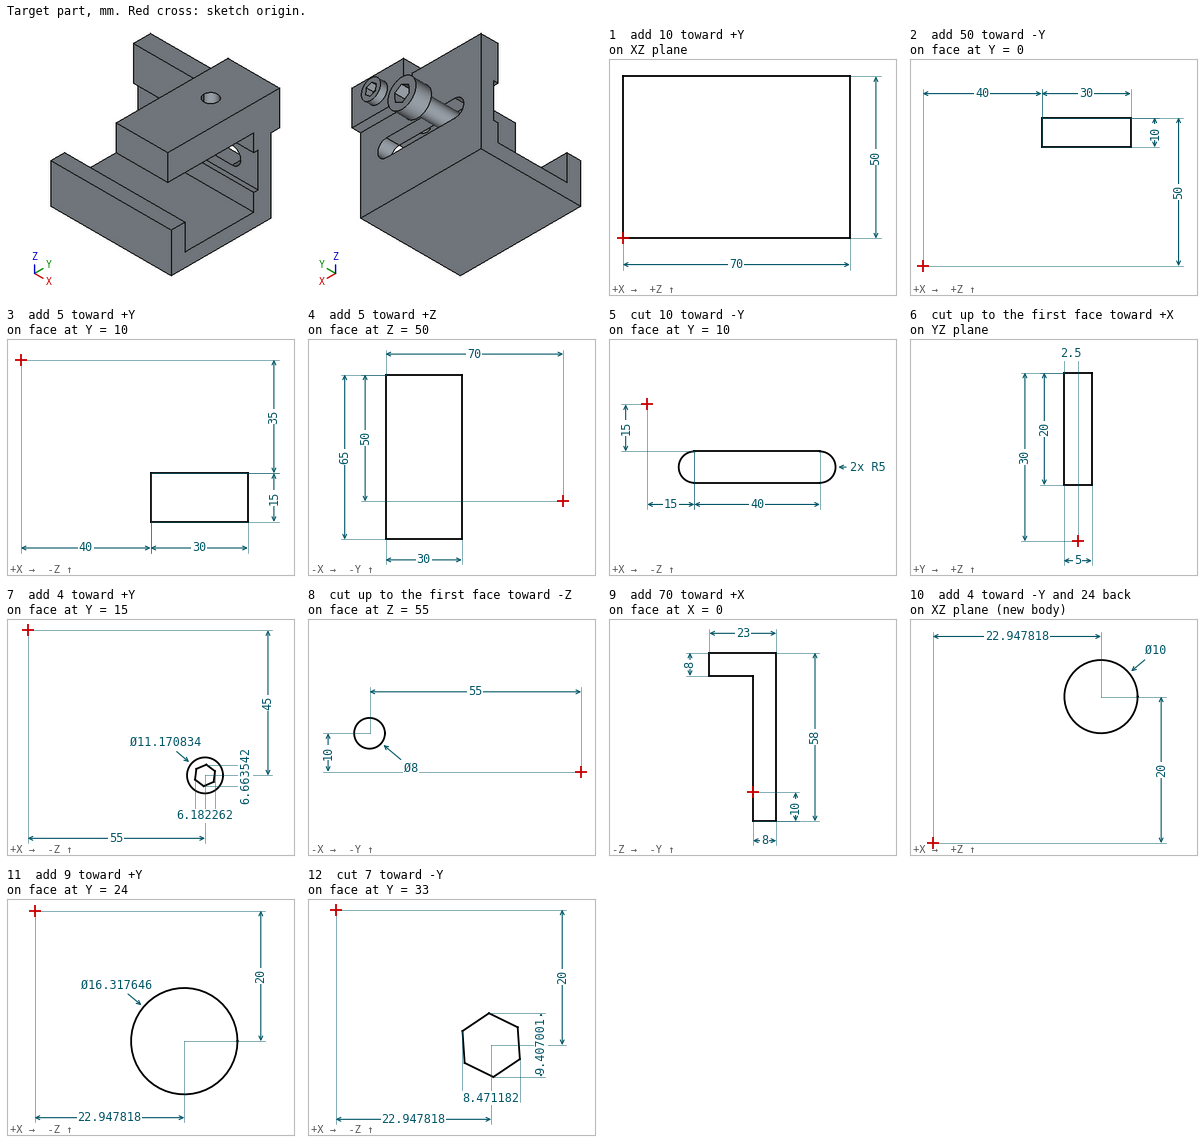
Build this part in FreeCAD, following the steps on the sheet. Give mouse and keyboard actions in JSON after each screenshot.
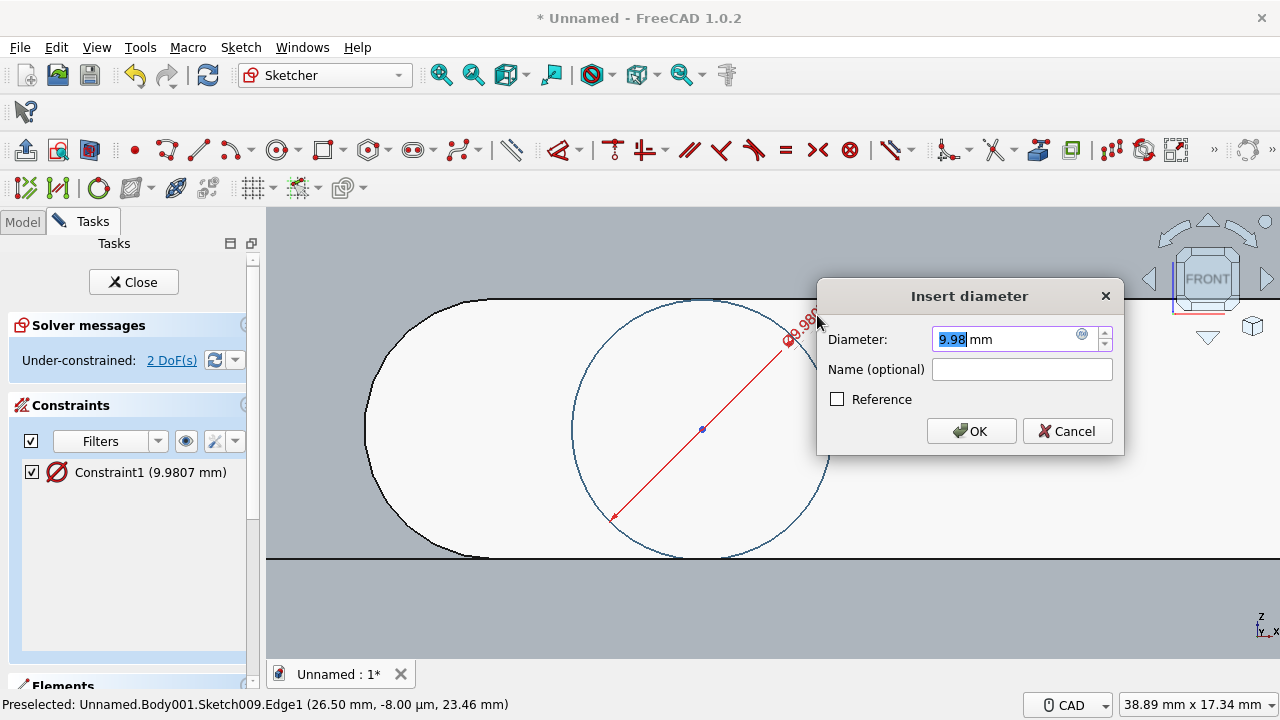
{"action": "type", "text": "10"}
{"action": "key", "text": "Return"}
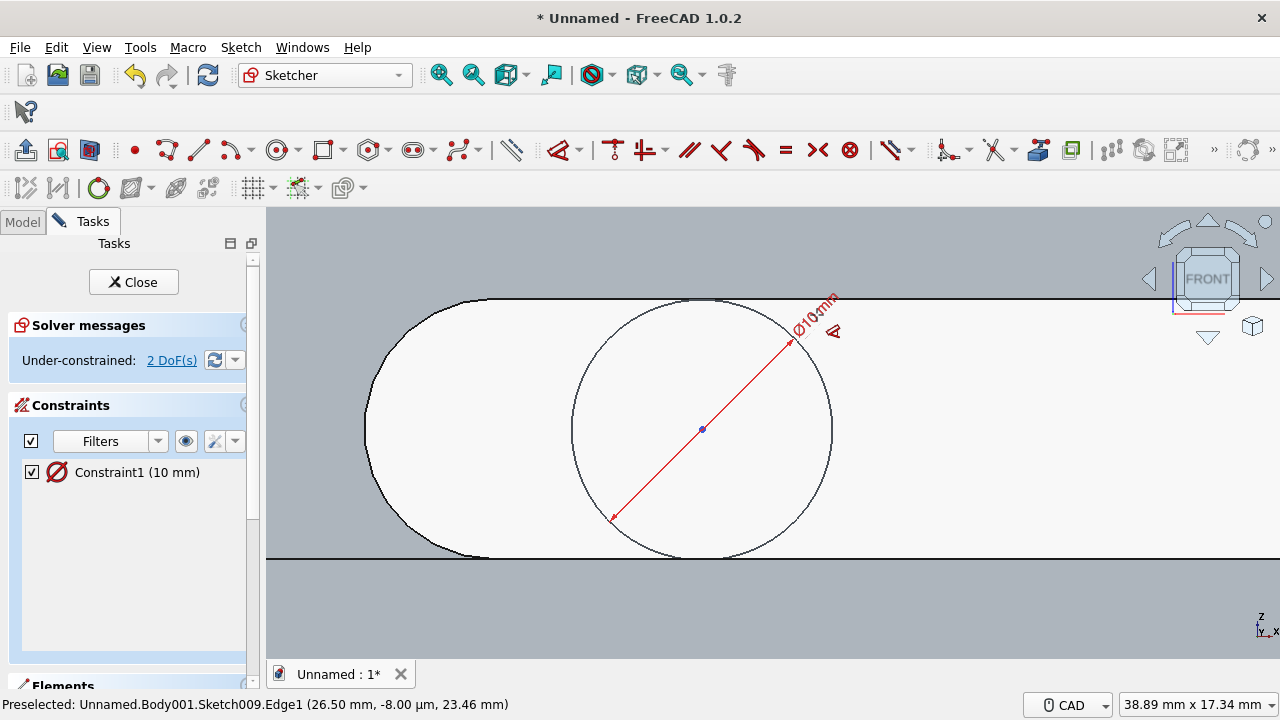
{"action": "left_click", "coordinate": [702, 430]}
{"action": "left_click", "coordinate": [736, 531]}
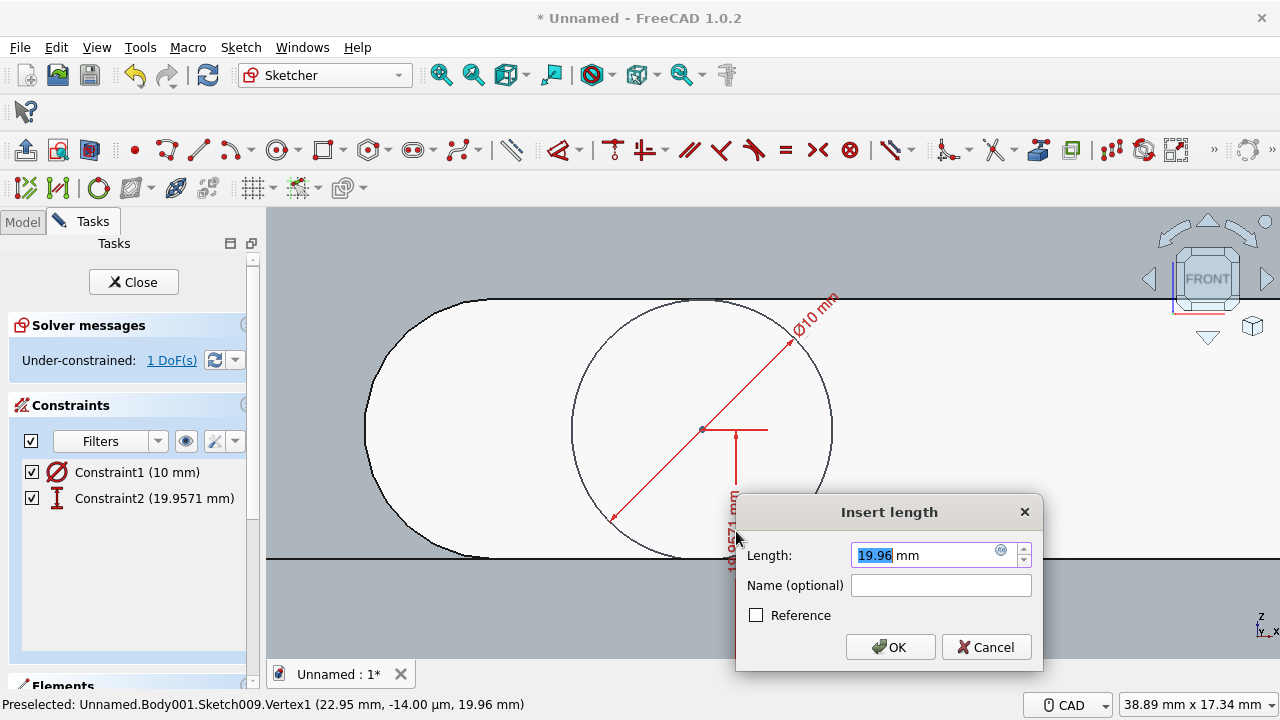
{"action": "type", "text": "20"}
{"action": "key", "text": "Return"}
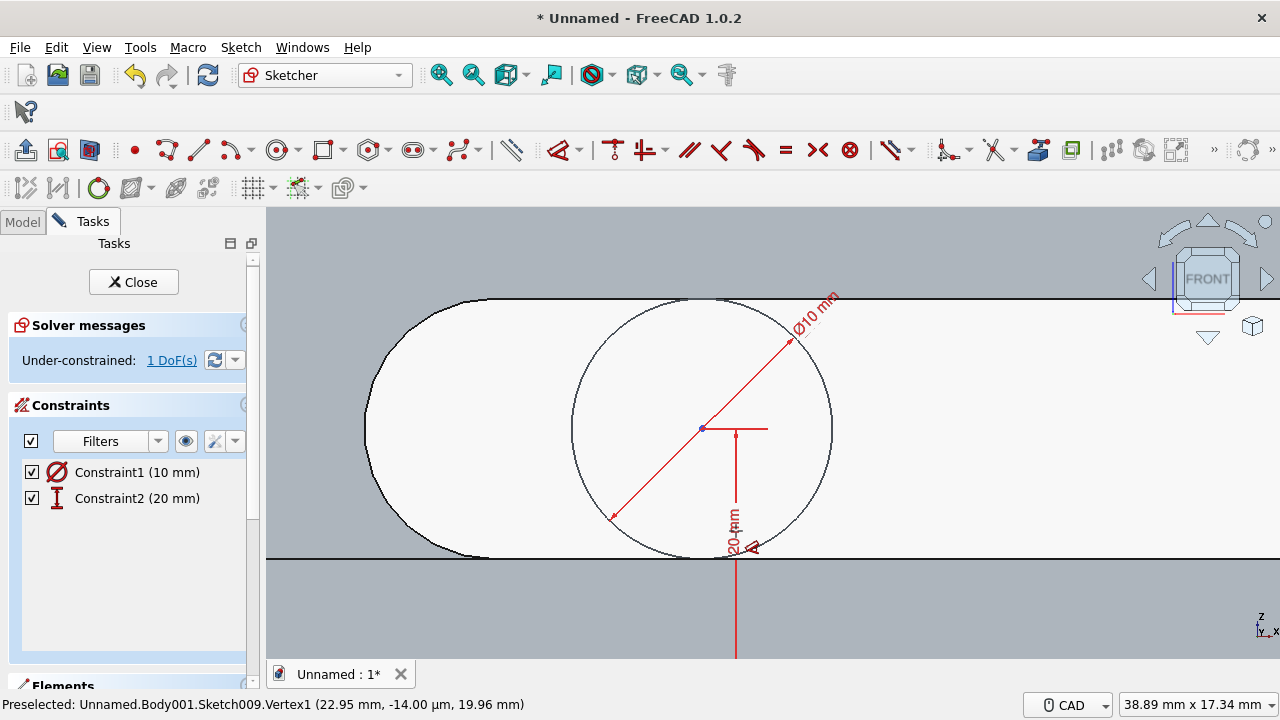
{"action": "left_click", "coordinate": [702, 429]}
{"action": "left_click", "coordinate": [498, 395]}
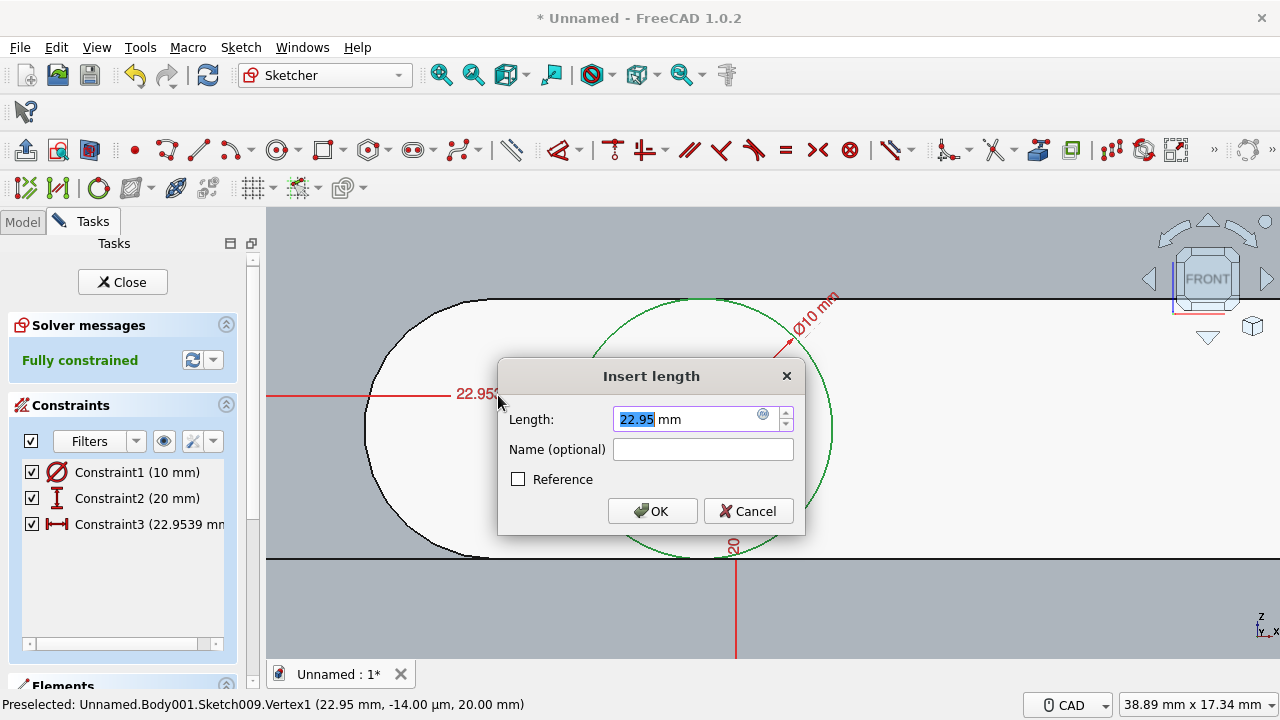
{"action": "type", "text": "22.947818"}
{"action": "key", "text": "Return"}
{"action": "key", "text": "Escape"}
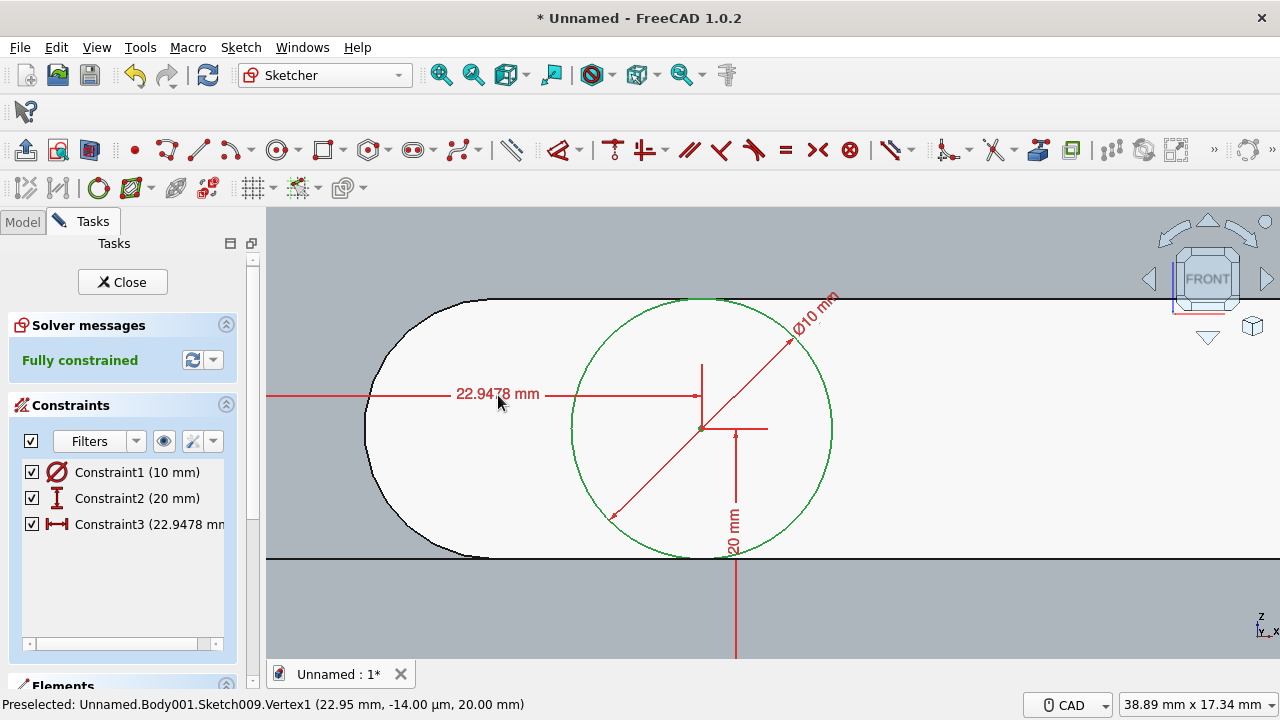
{"action": "left_click", "coordinate": [123, 282]}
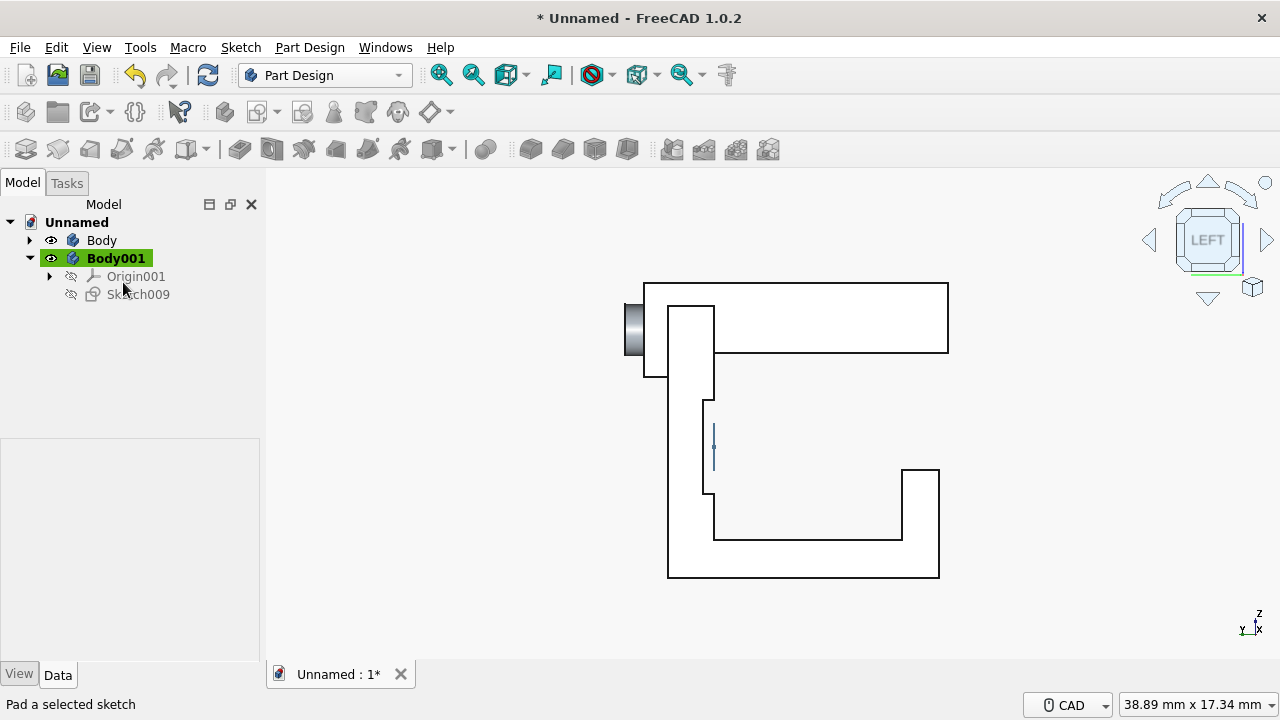
{"action": "left_click", "coordinate": [26, 150]}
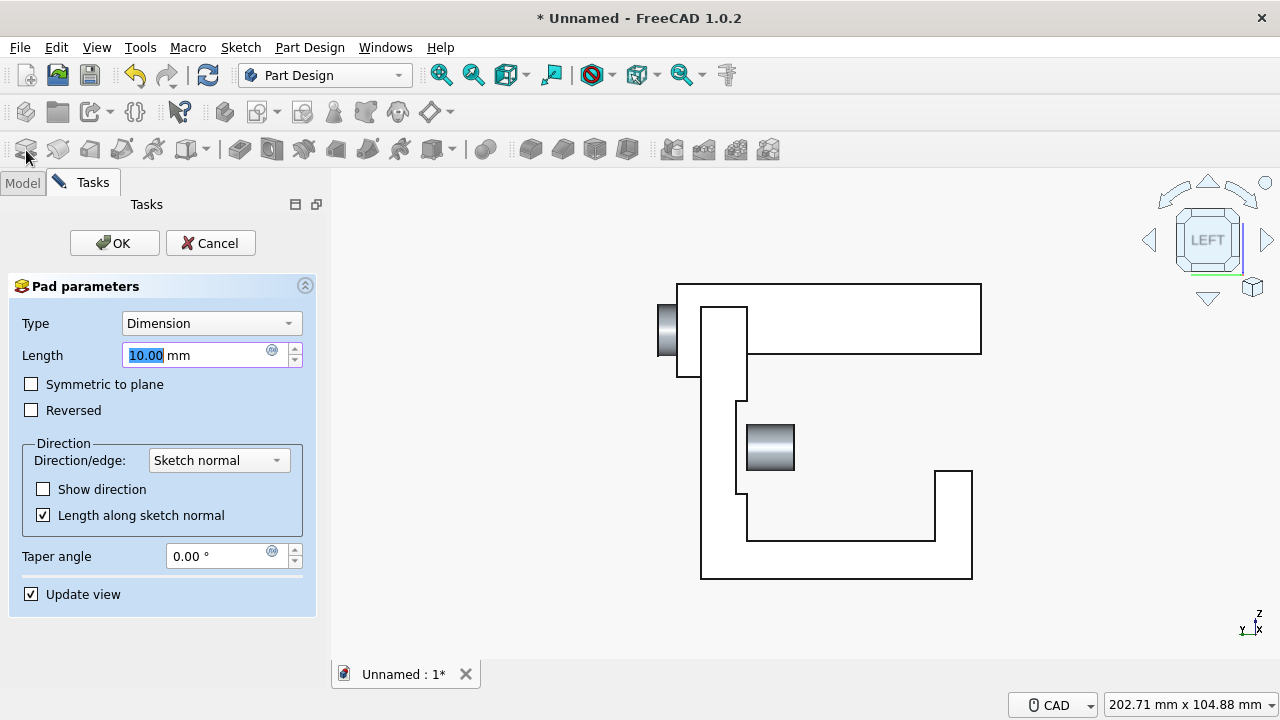
{"action": "left_click", "coordinate": [212, 324]}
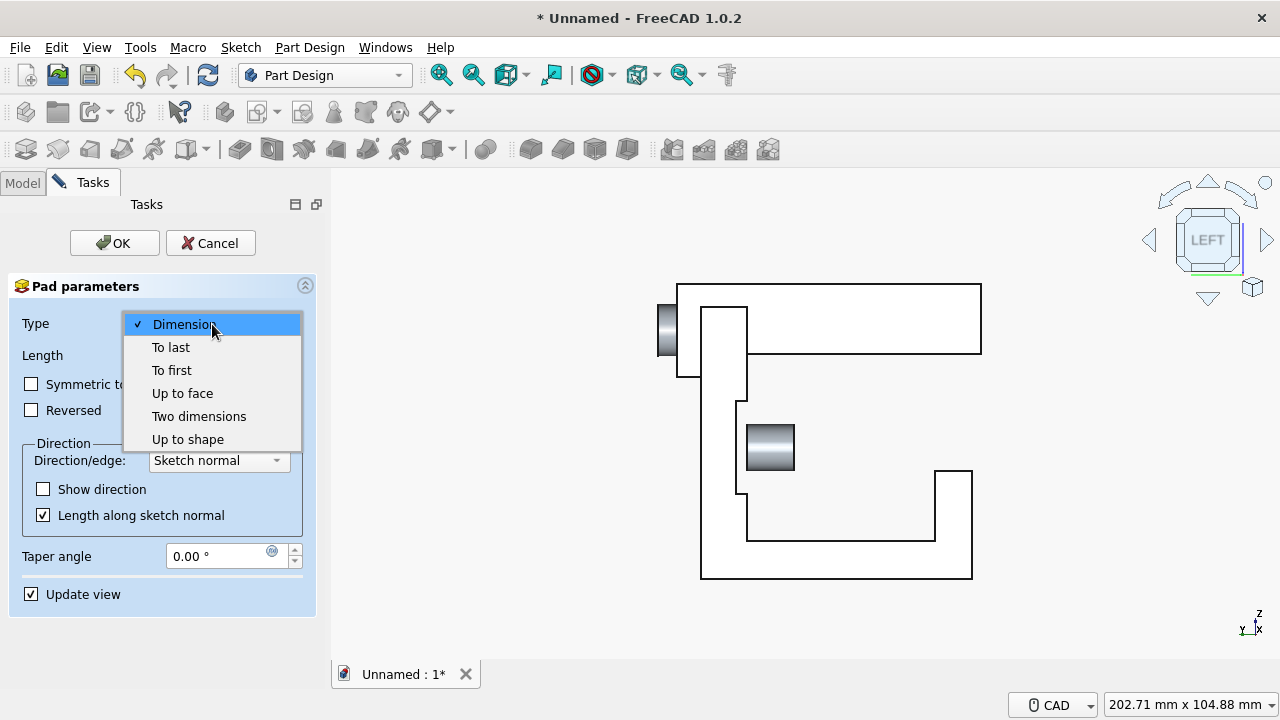
{"action": "left_click", "coordinate": [212, 416]}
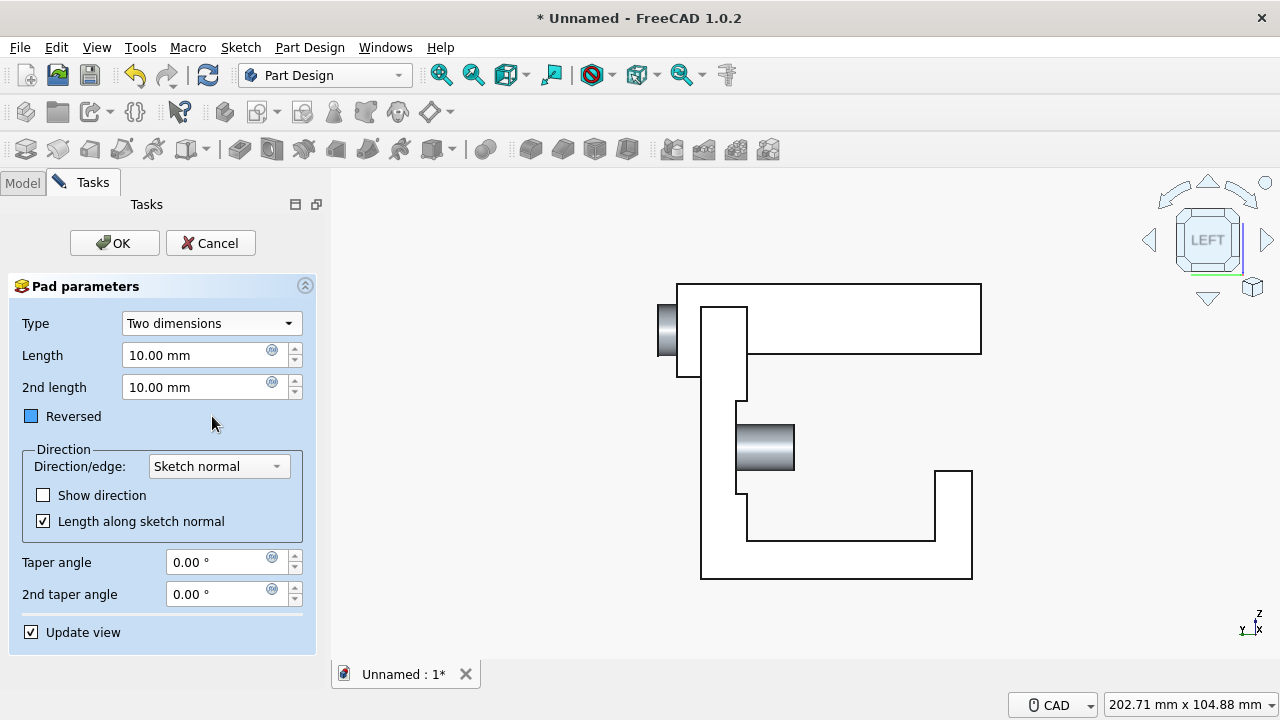
{"action": "triple_click", "coordinate": [204, 355]}